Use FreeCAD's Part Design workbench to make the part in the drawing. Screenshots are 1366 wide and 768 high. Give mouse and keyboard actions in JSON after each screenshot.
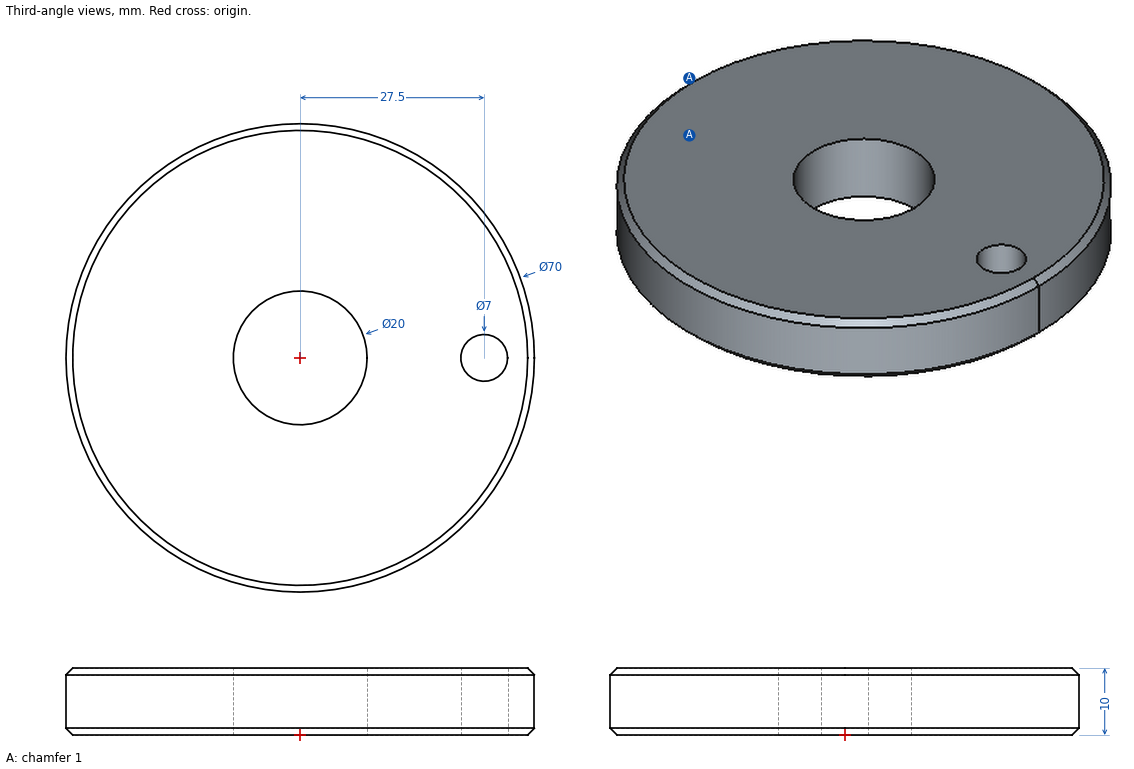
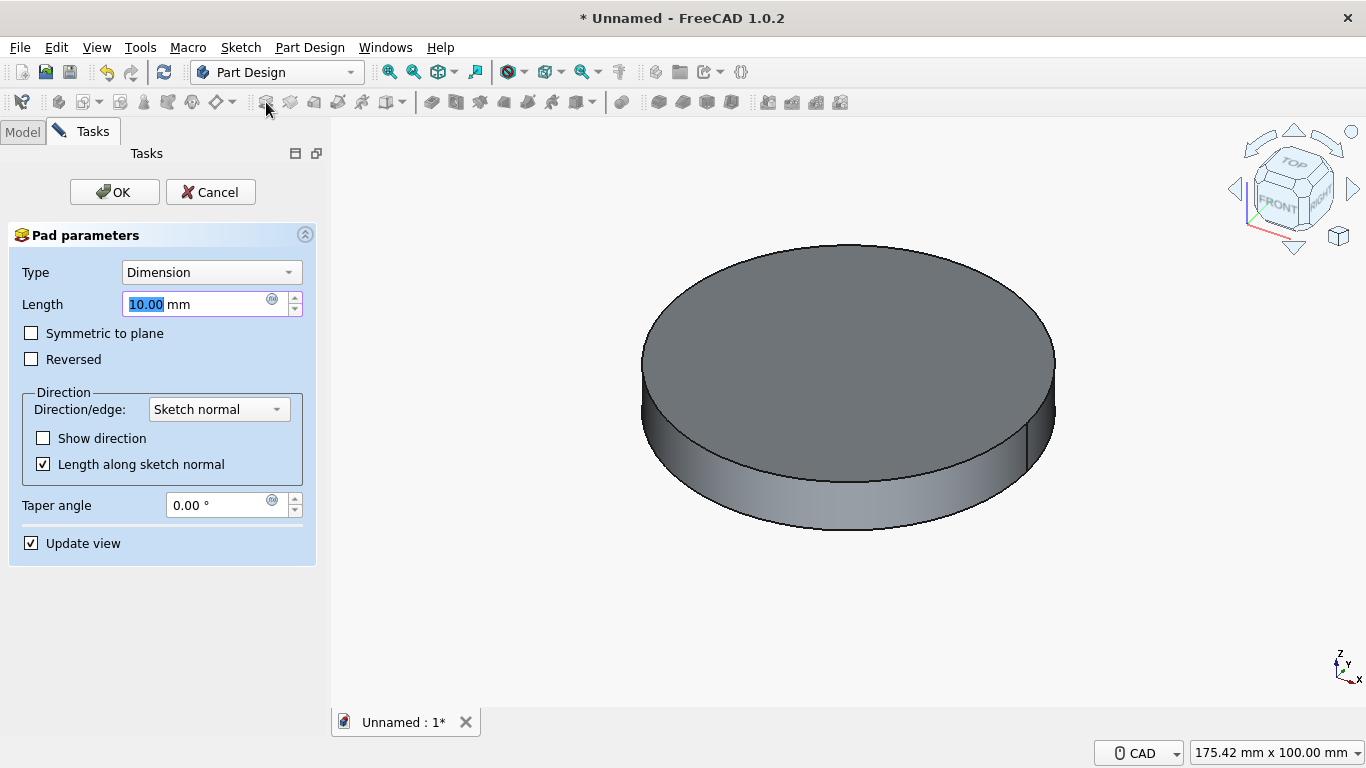
{"action": "type", "text": "10"}
{"action": "key", "text": "Tab"}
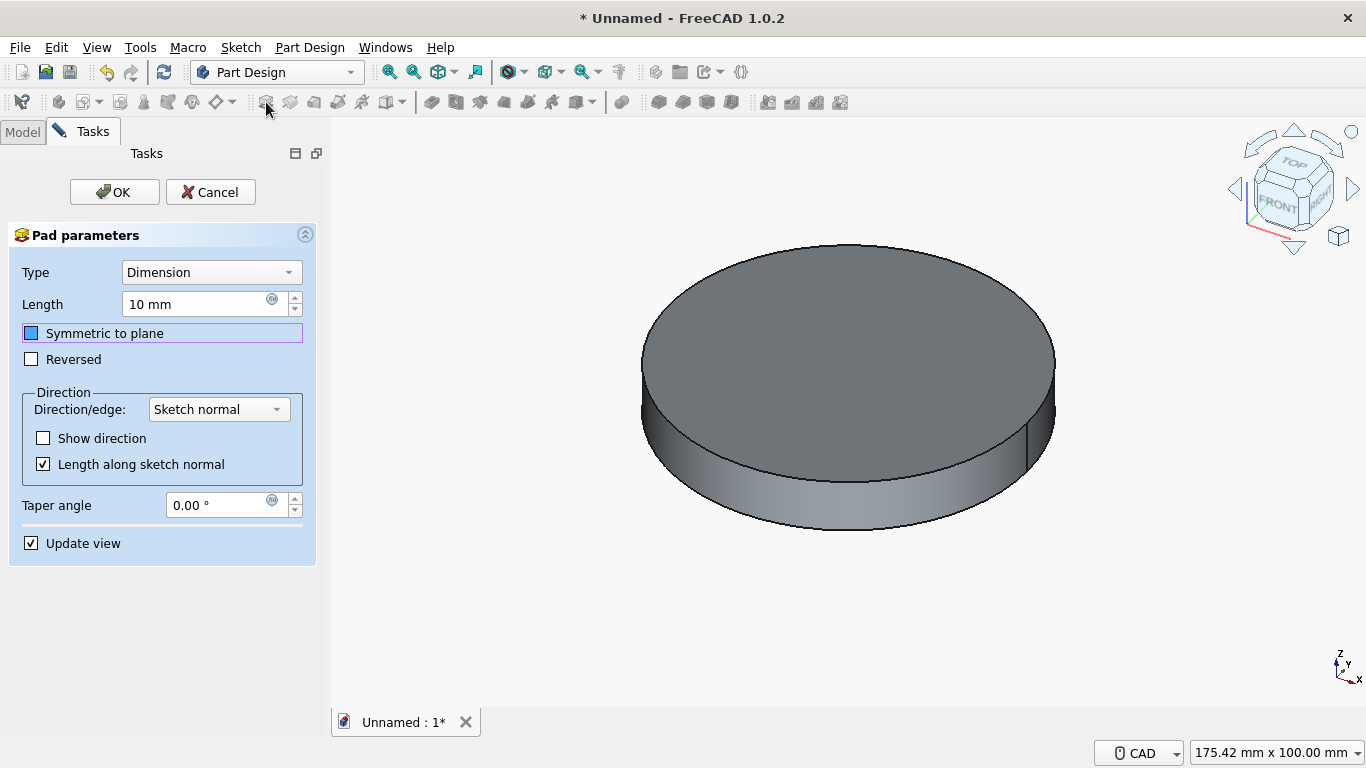
{"action": "left_click", "coordinate": [115, 192]}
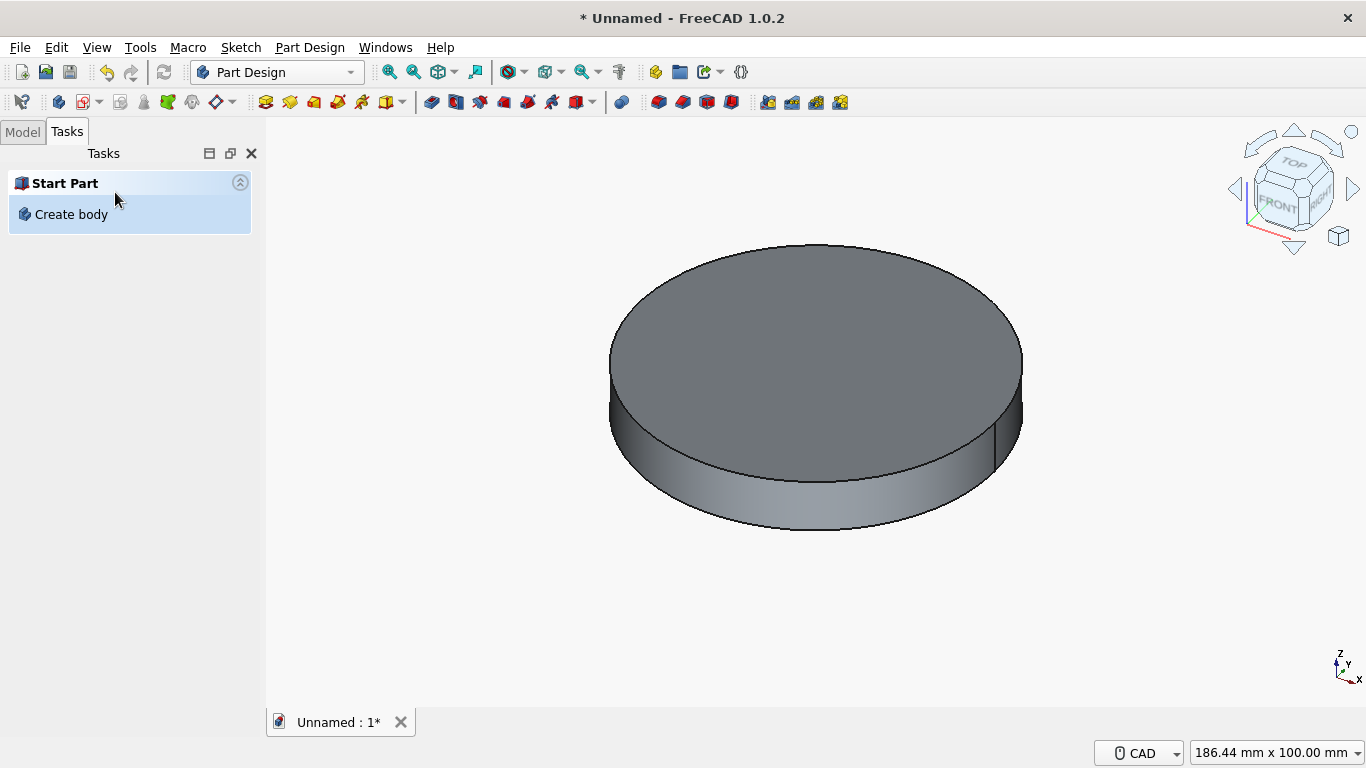
{"action": "left_click", "coordinate": [611, 375]}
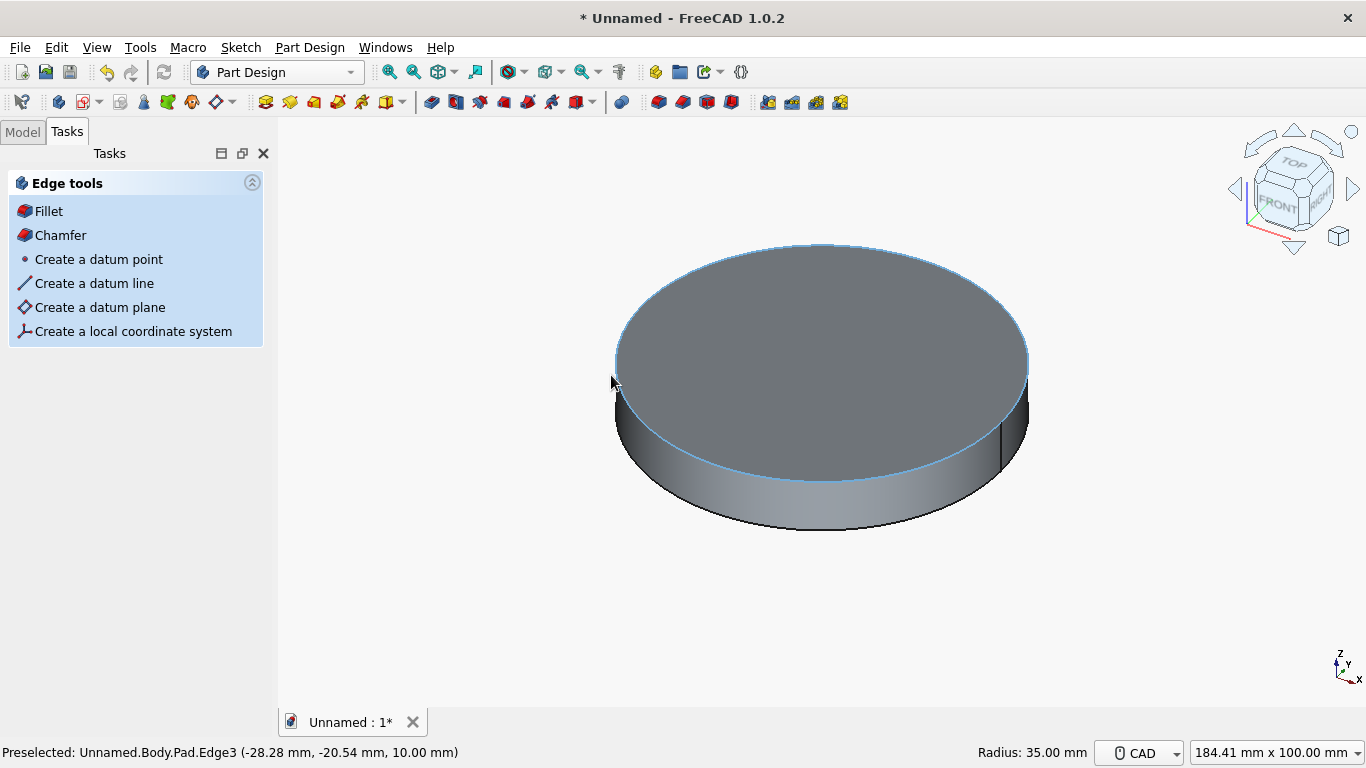
{"action": "key", "text": "0"}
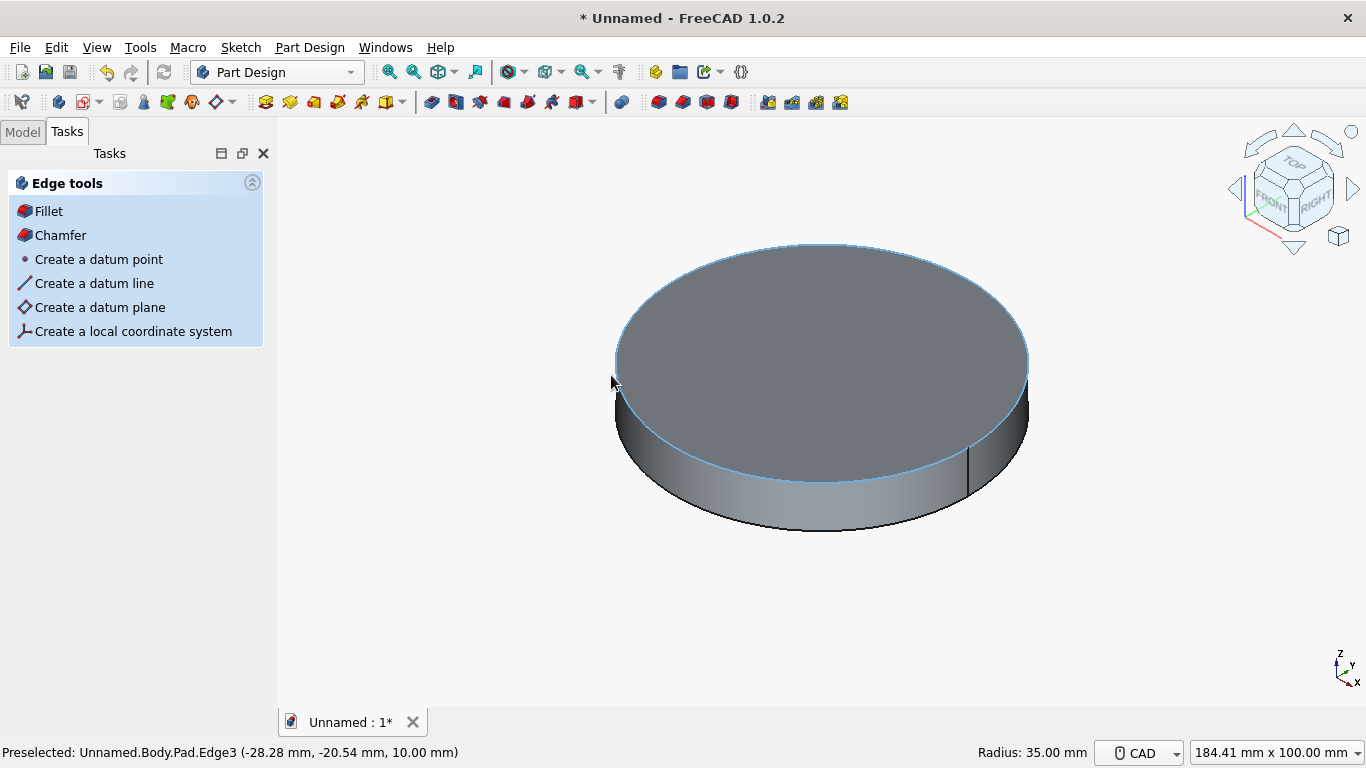
{"action": "key", "text": "2"}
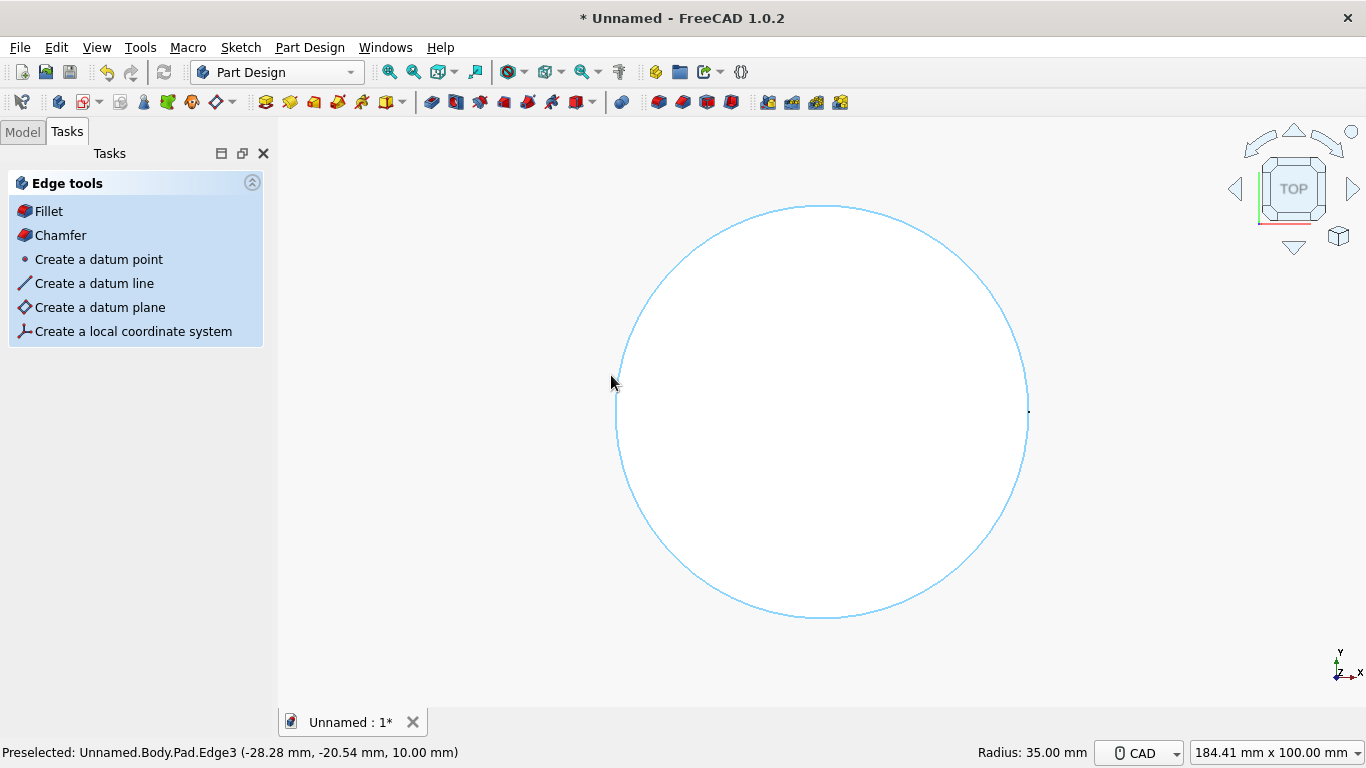
{"action": "key", "text": "1"}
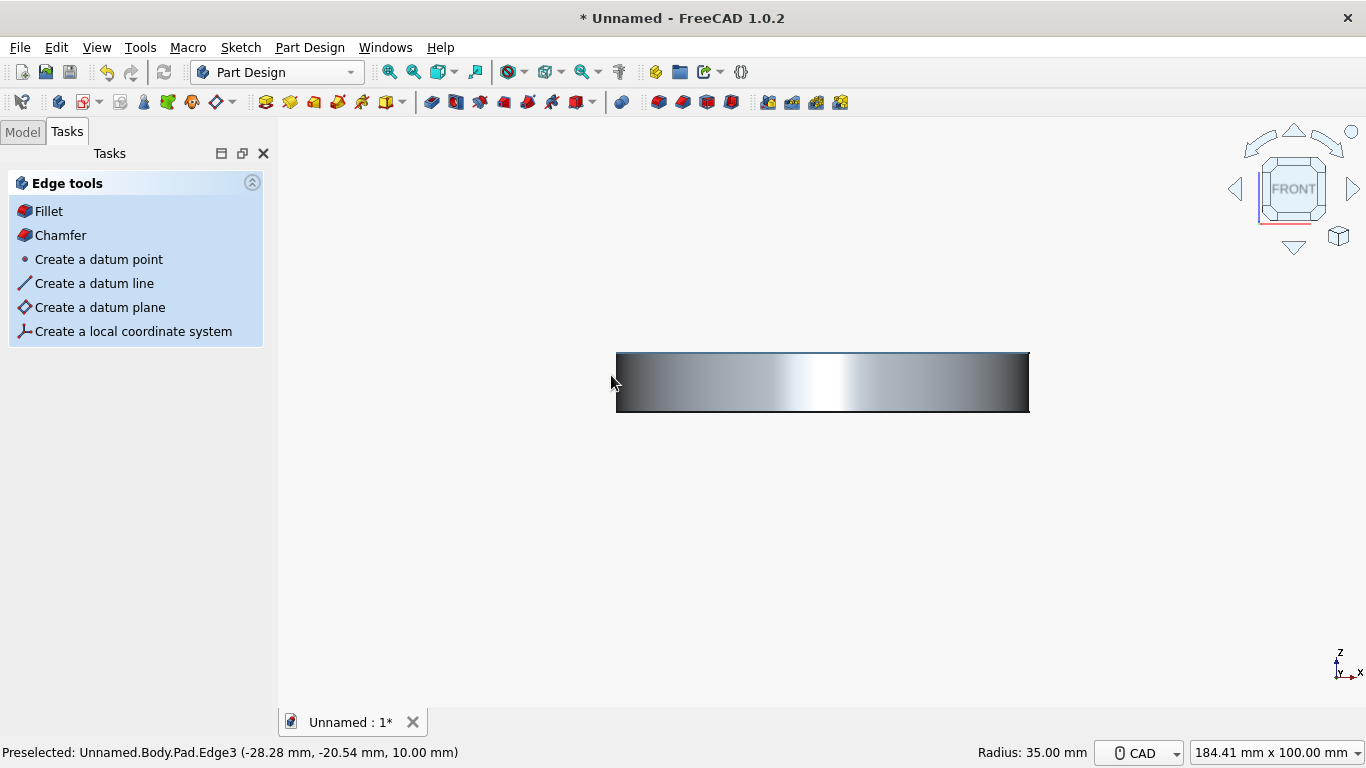
{"action": "left_click", "coordinate": [390, 72]}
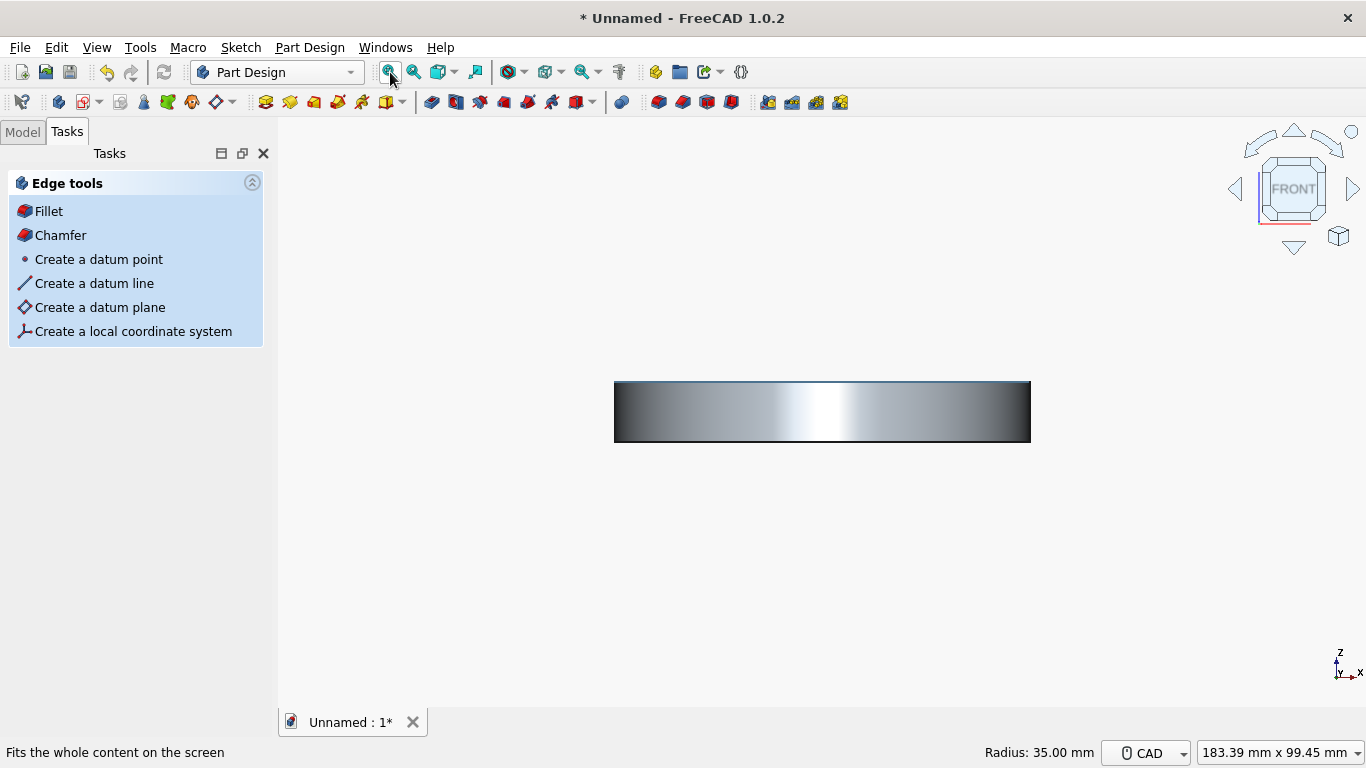
{"action": "left_click", "coordinate": [654, 441], "text": "ctrl"}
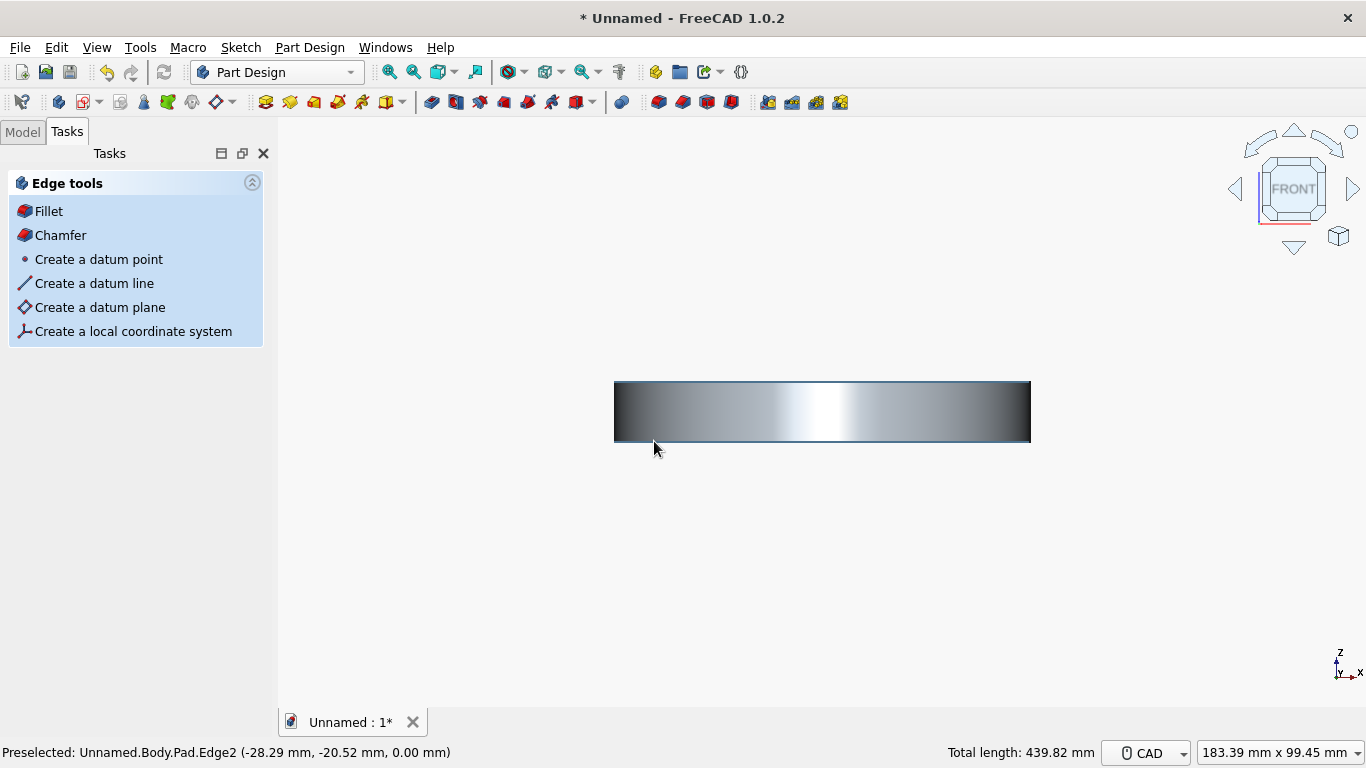
{"action": "left_click", "coordinate": [684, 102]}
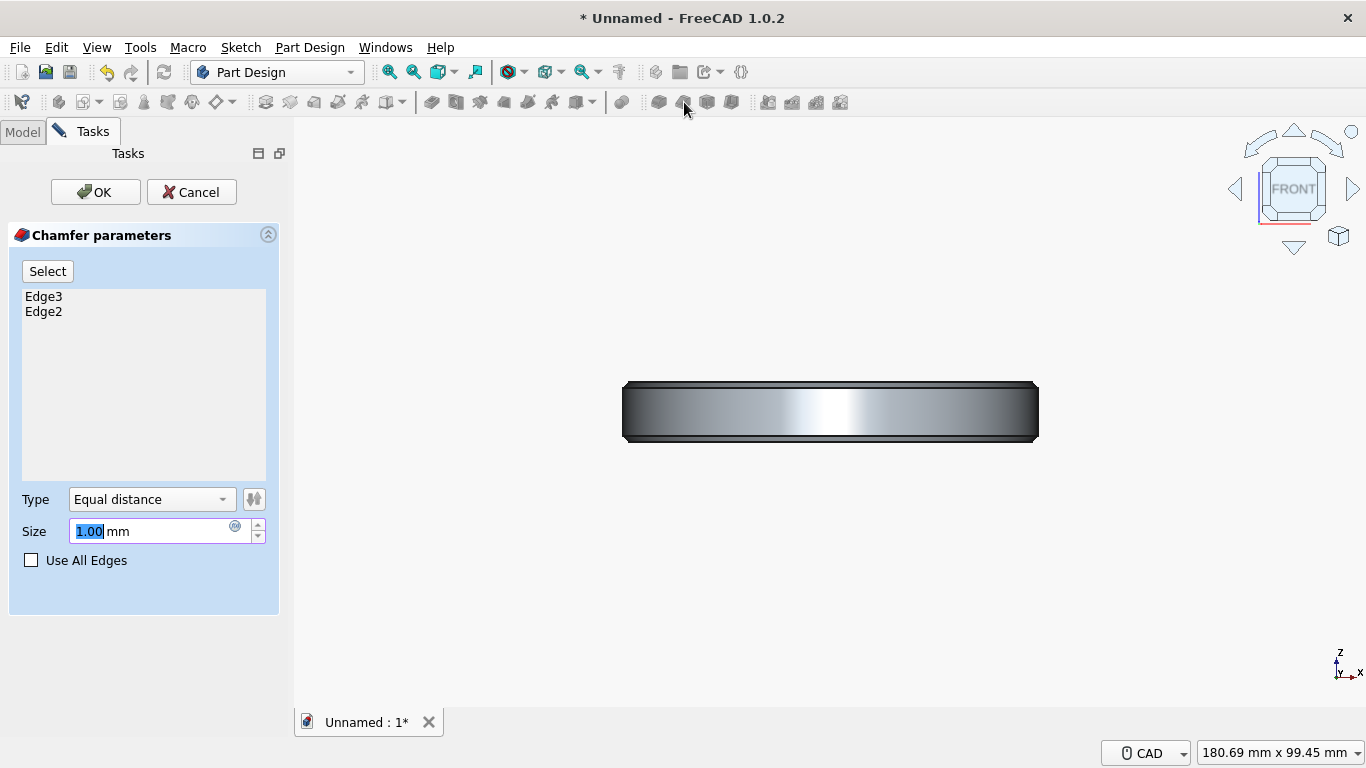
{"action": "type", "text": "1"}
{"action": "key", "text": "Tab"}